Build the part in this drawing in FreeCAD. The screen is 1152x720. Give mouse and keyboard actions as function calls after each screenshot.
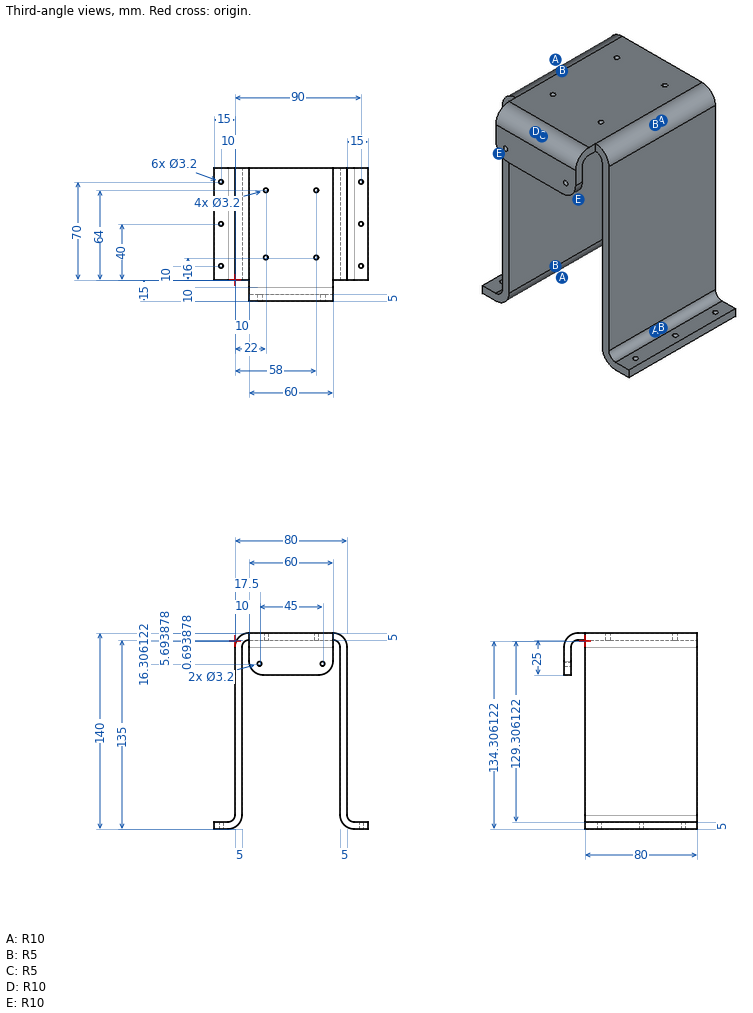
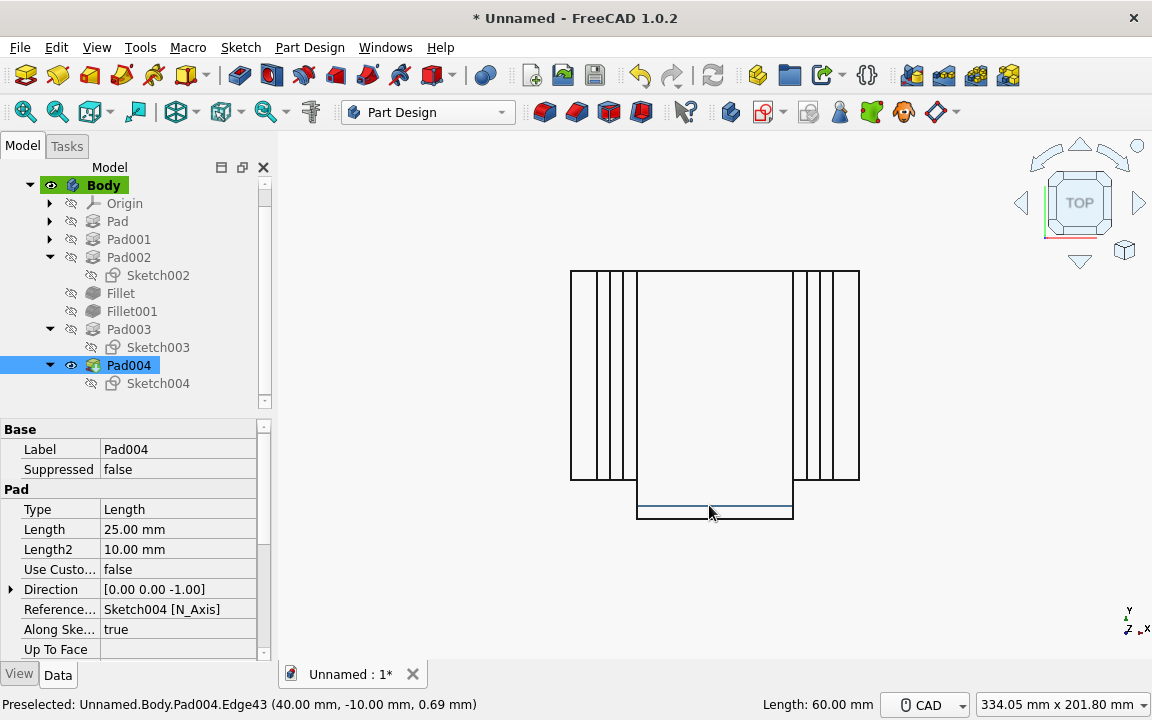
key(v)
key(1)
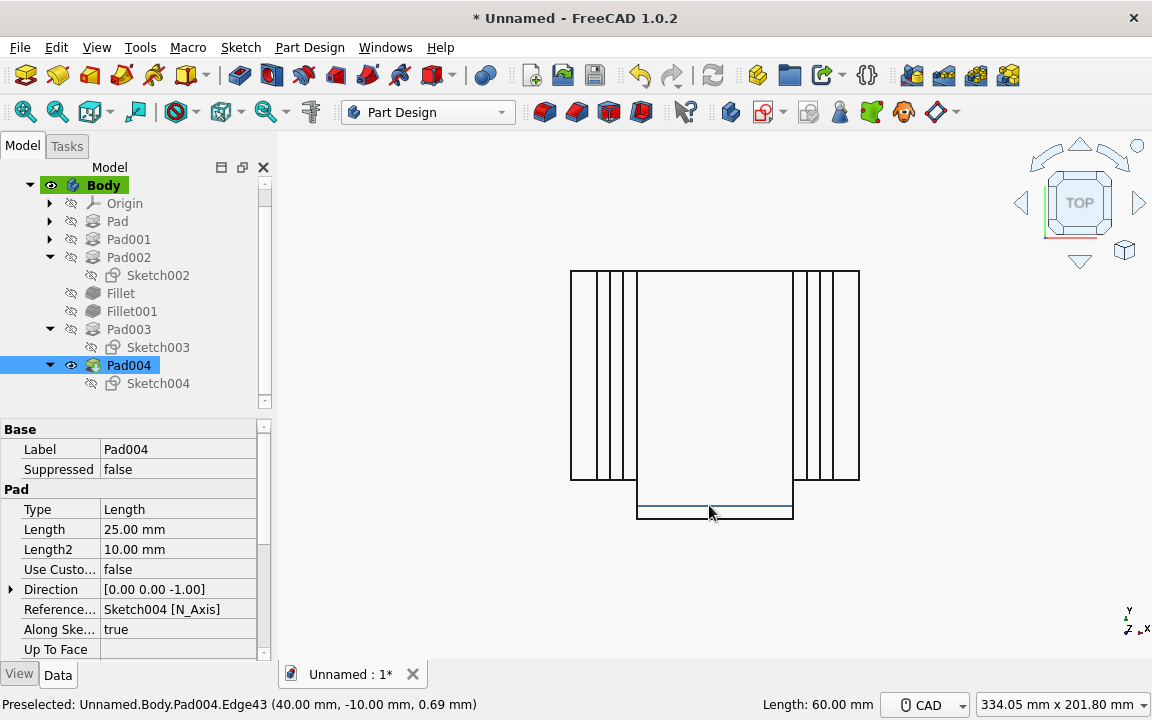
click(546, 112)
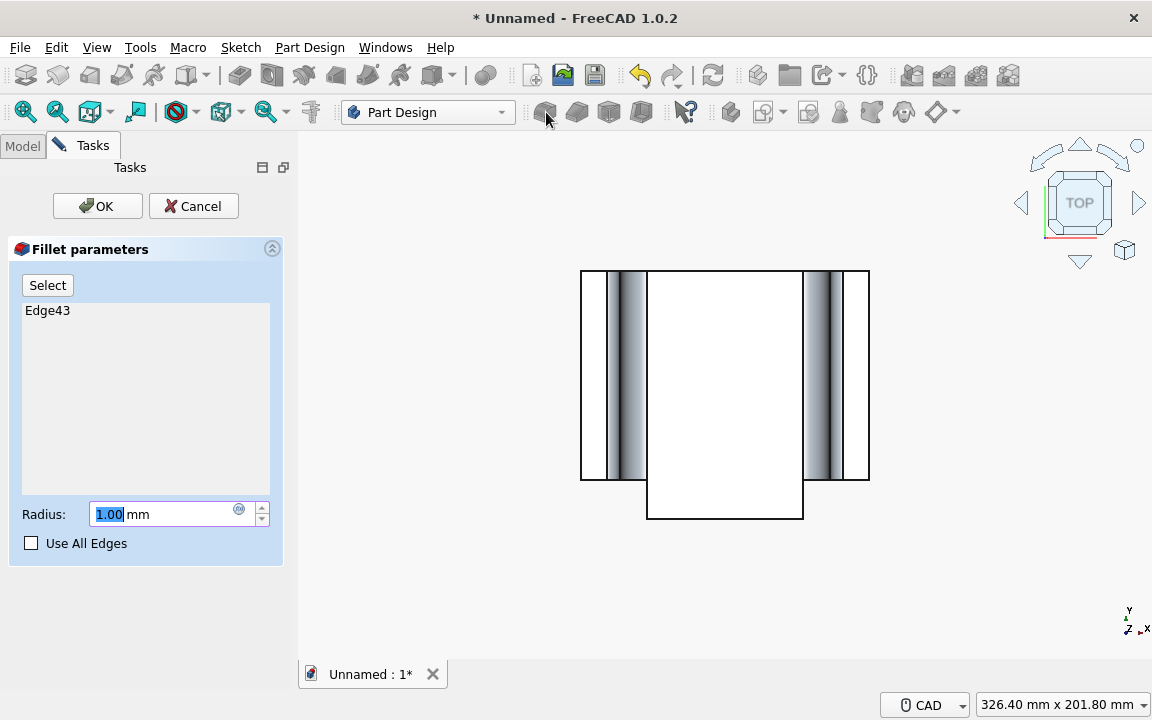
text(5)
key(Tab)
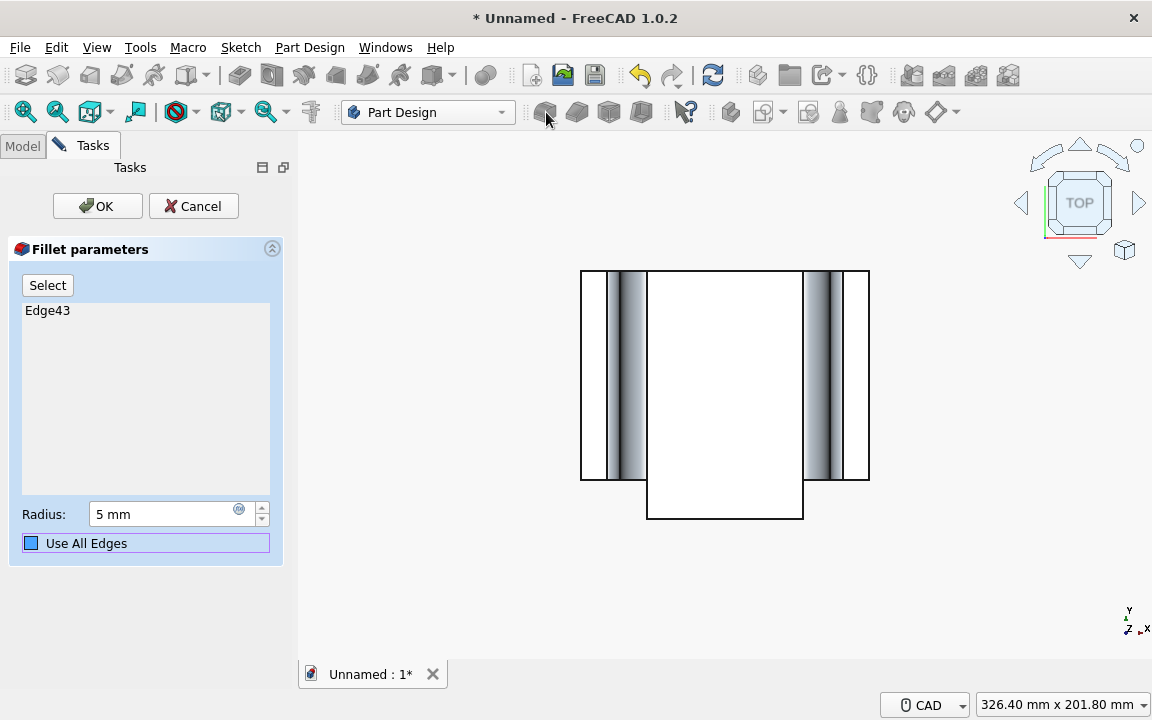
click(98, 206)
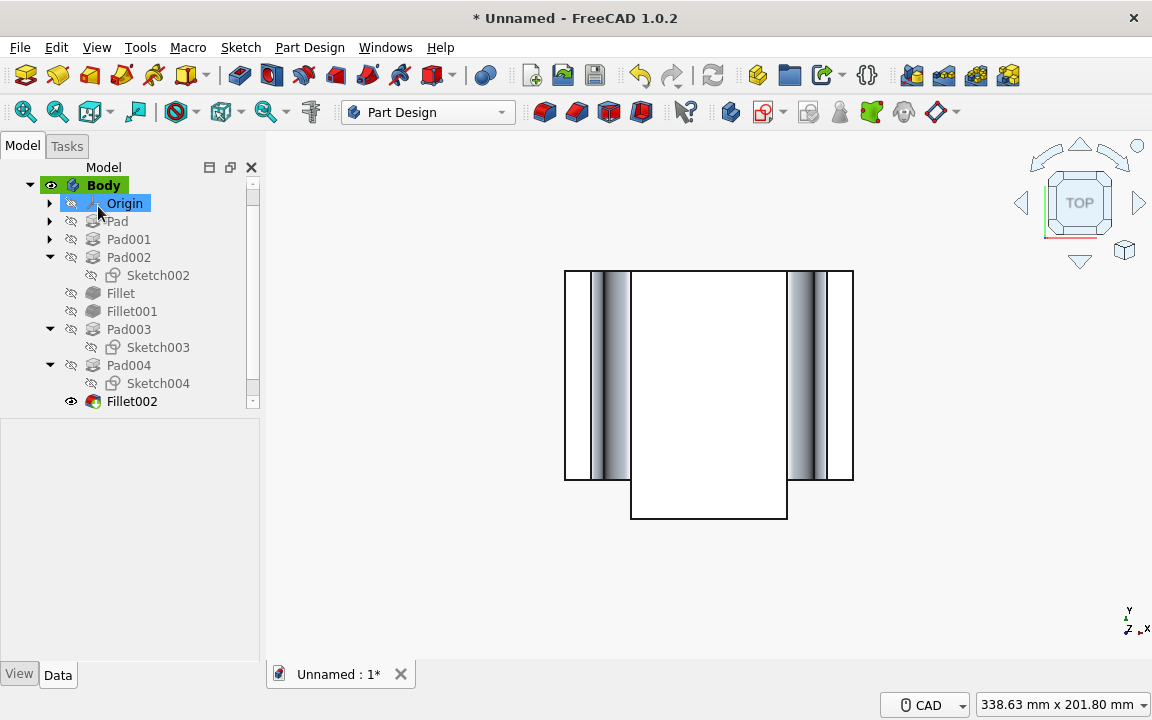
key(0)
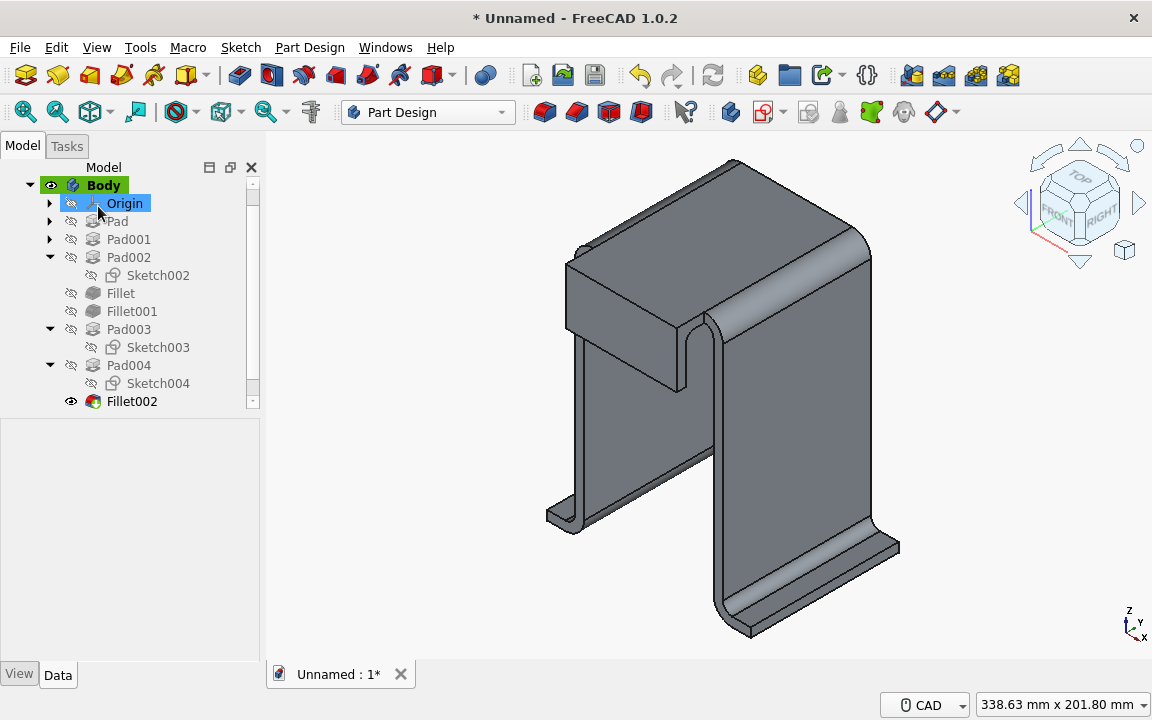
click(621, 295)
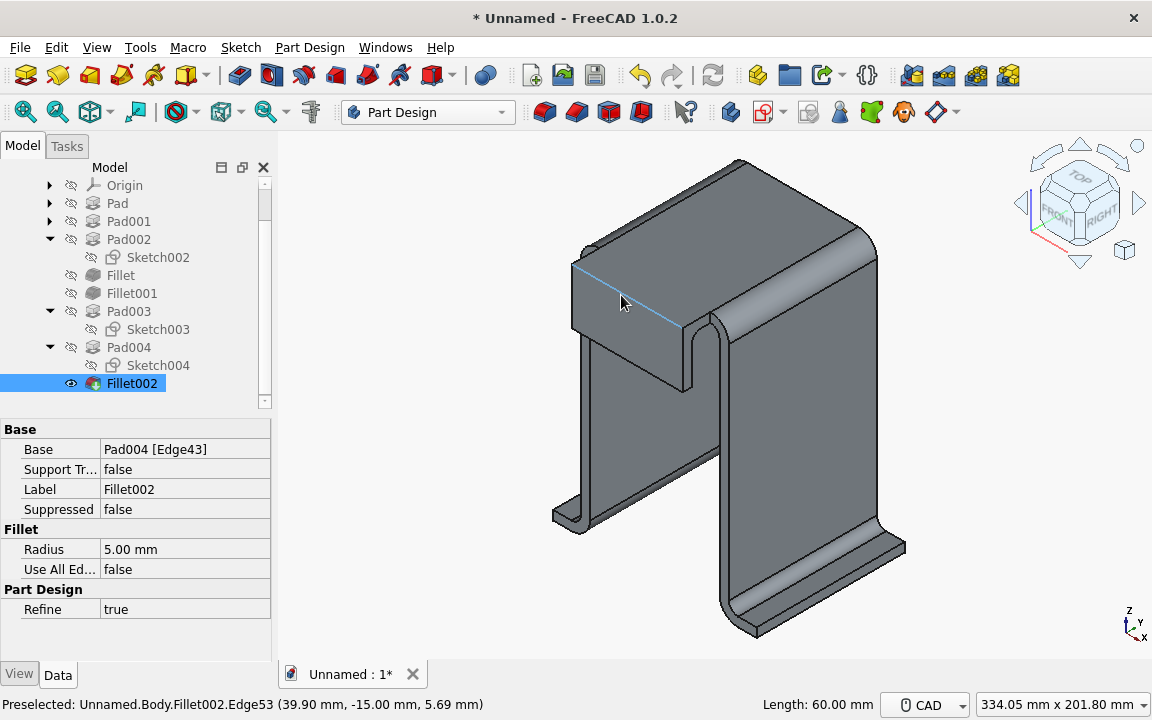
click(546, 112)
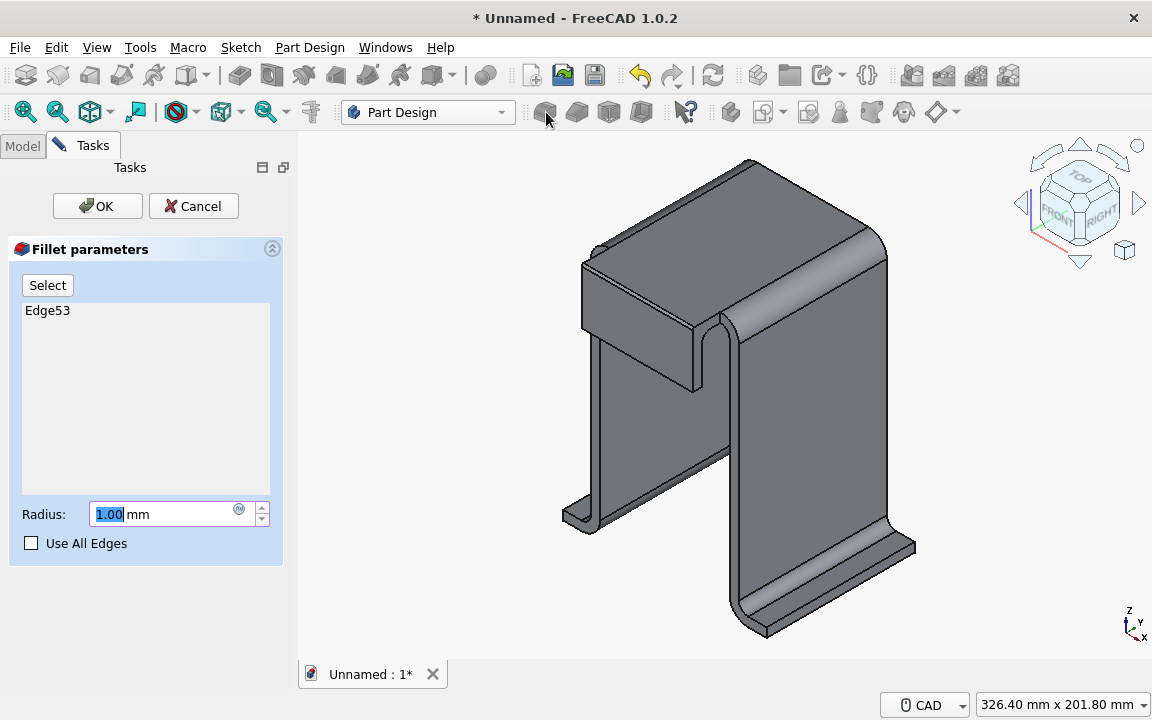
text(10)
key(Tab)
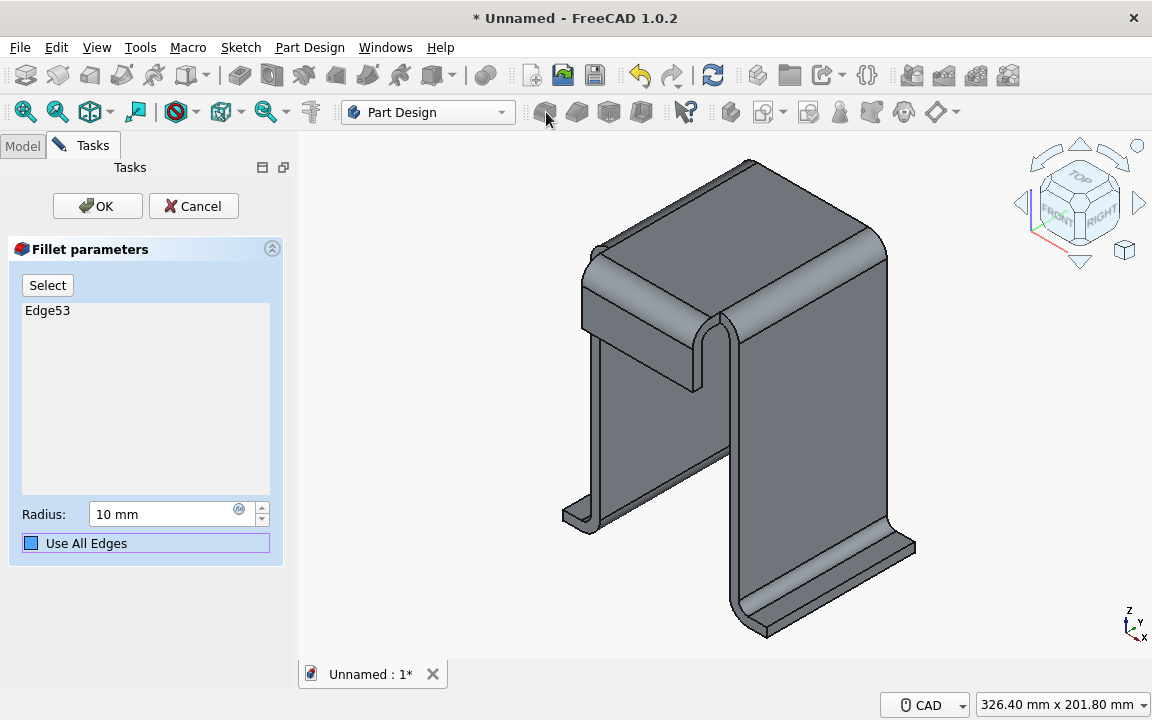
click(98, 206)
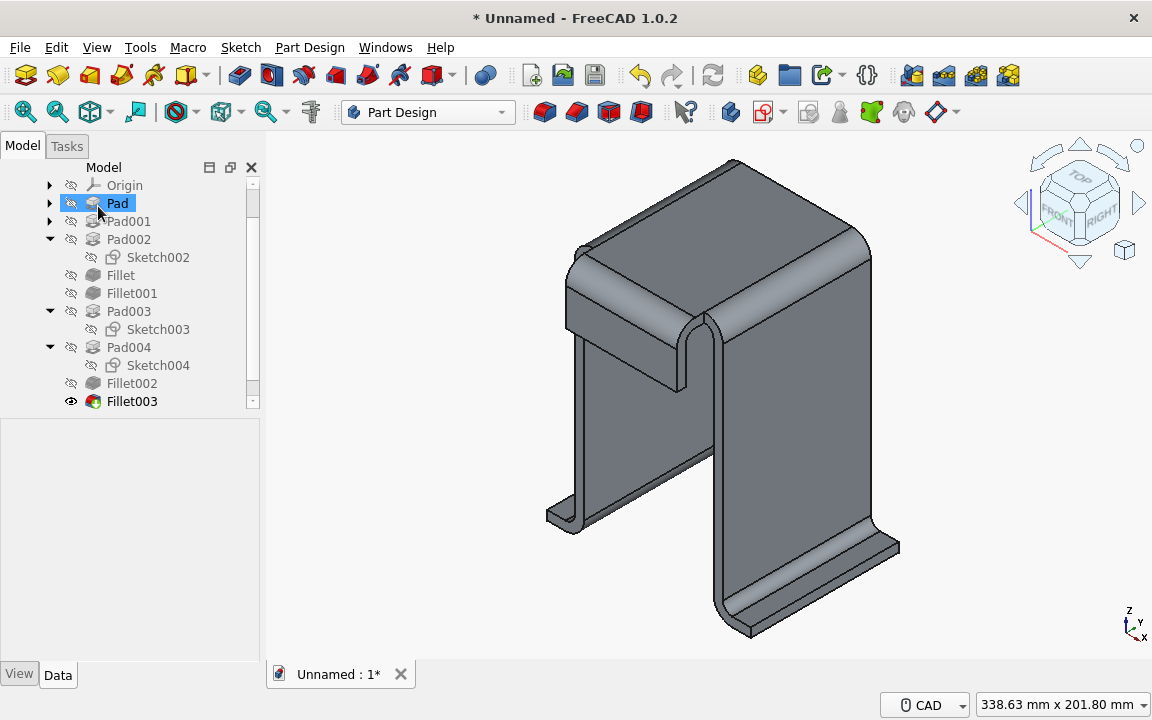
click(653, 356)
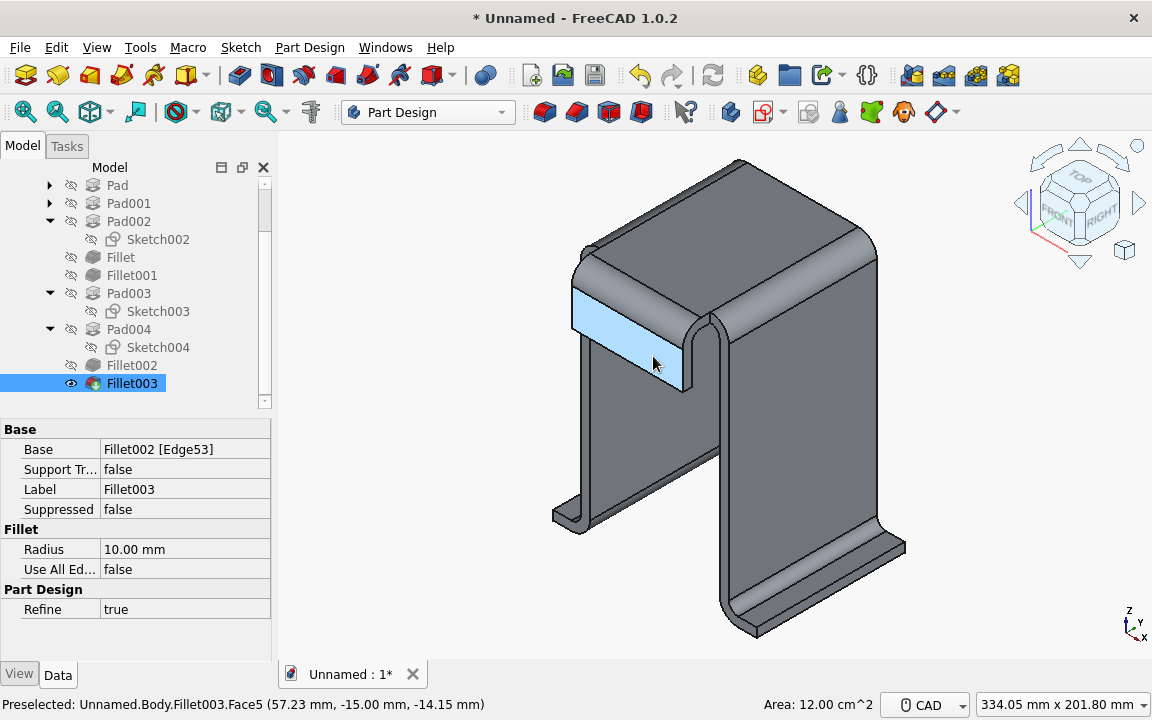
click(764, 112)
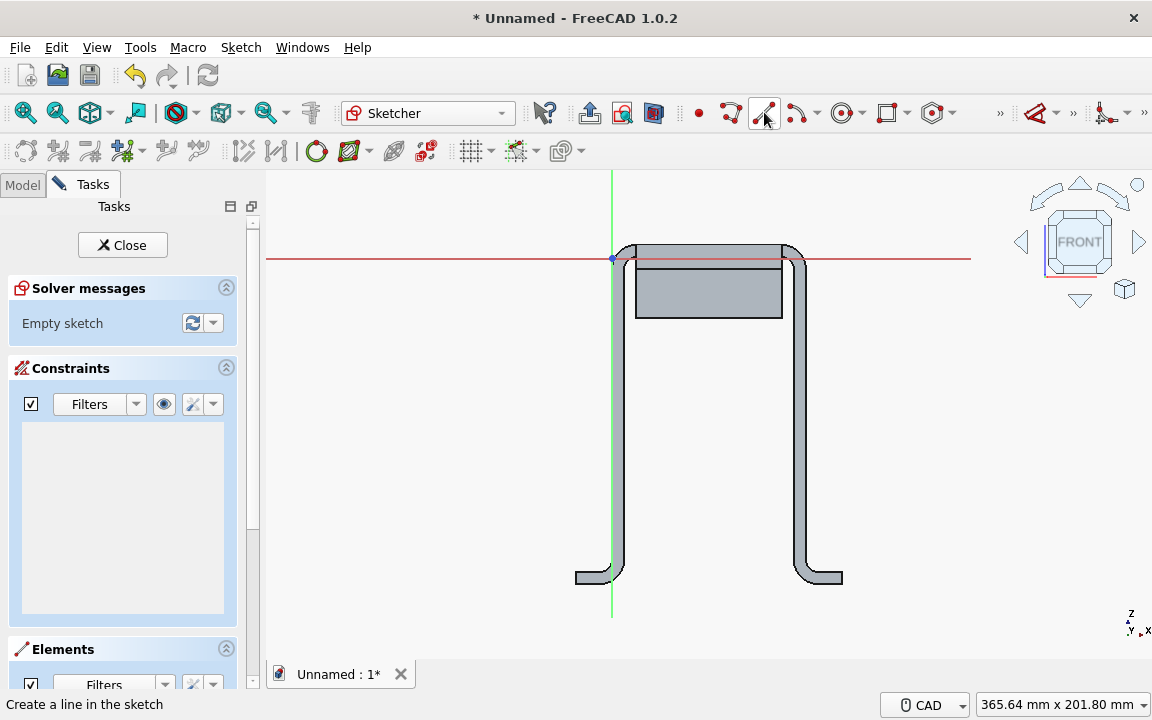
scroll(711, 223, up, 6)